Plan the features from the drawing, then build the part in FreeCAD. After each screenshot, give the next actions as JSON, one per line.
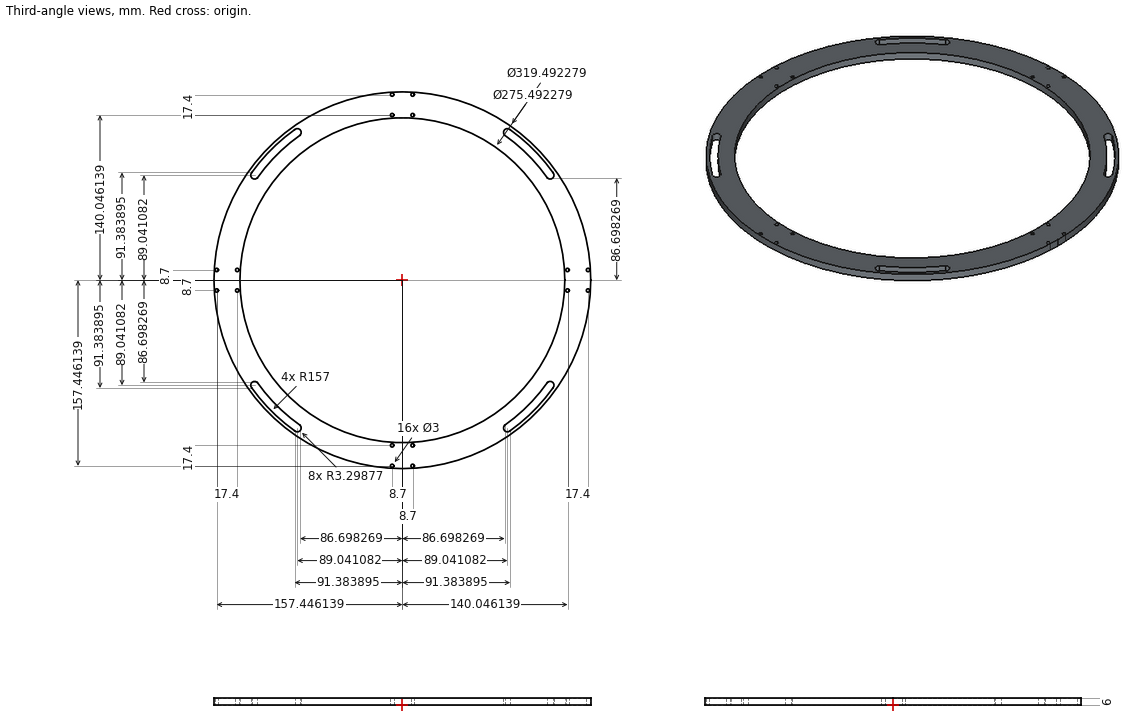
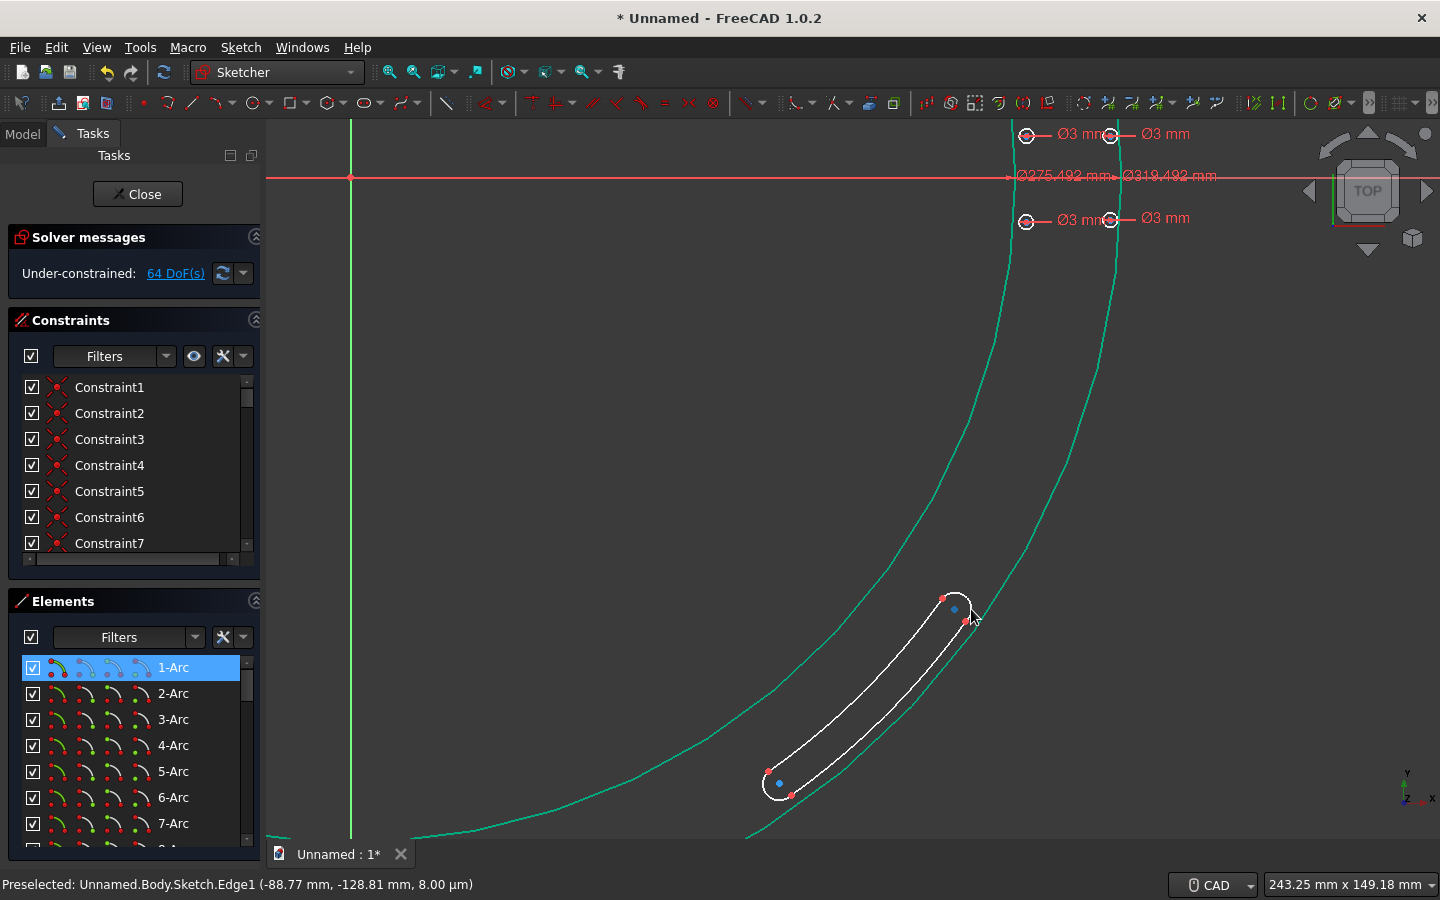
{"action": "left_click", "coordinate": [971, 607]}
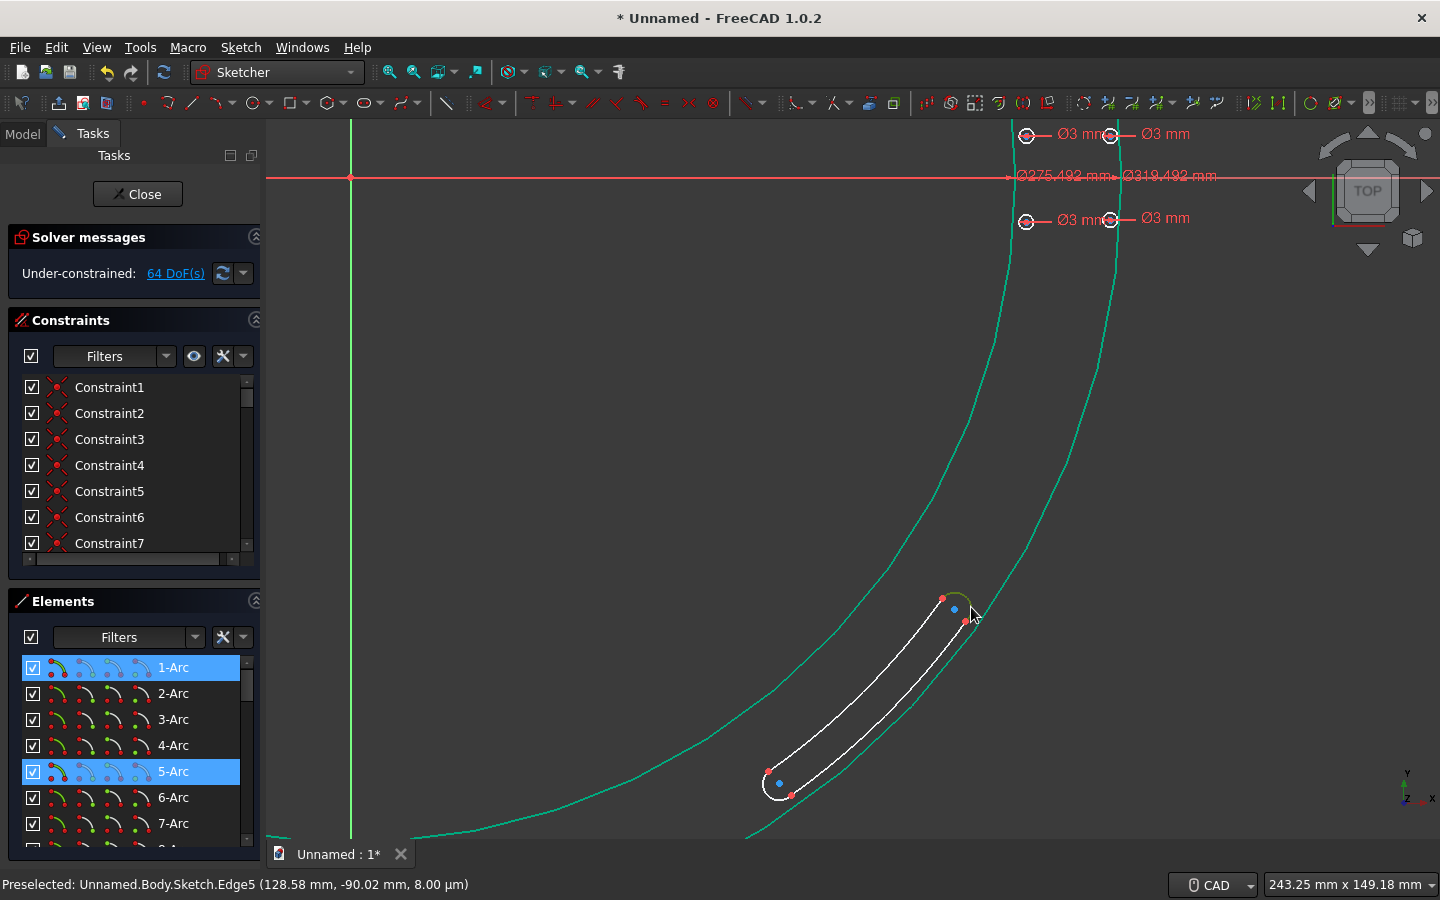
{"action": "scroll", "coordinate": [972, 609], "scroll_direction": "down", "scroll_amount": 6}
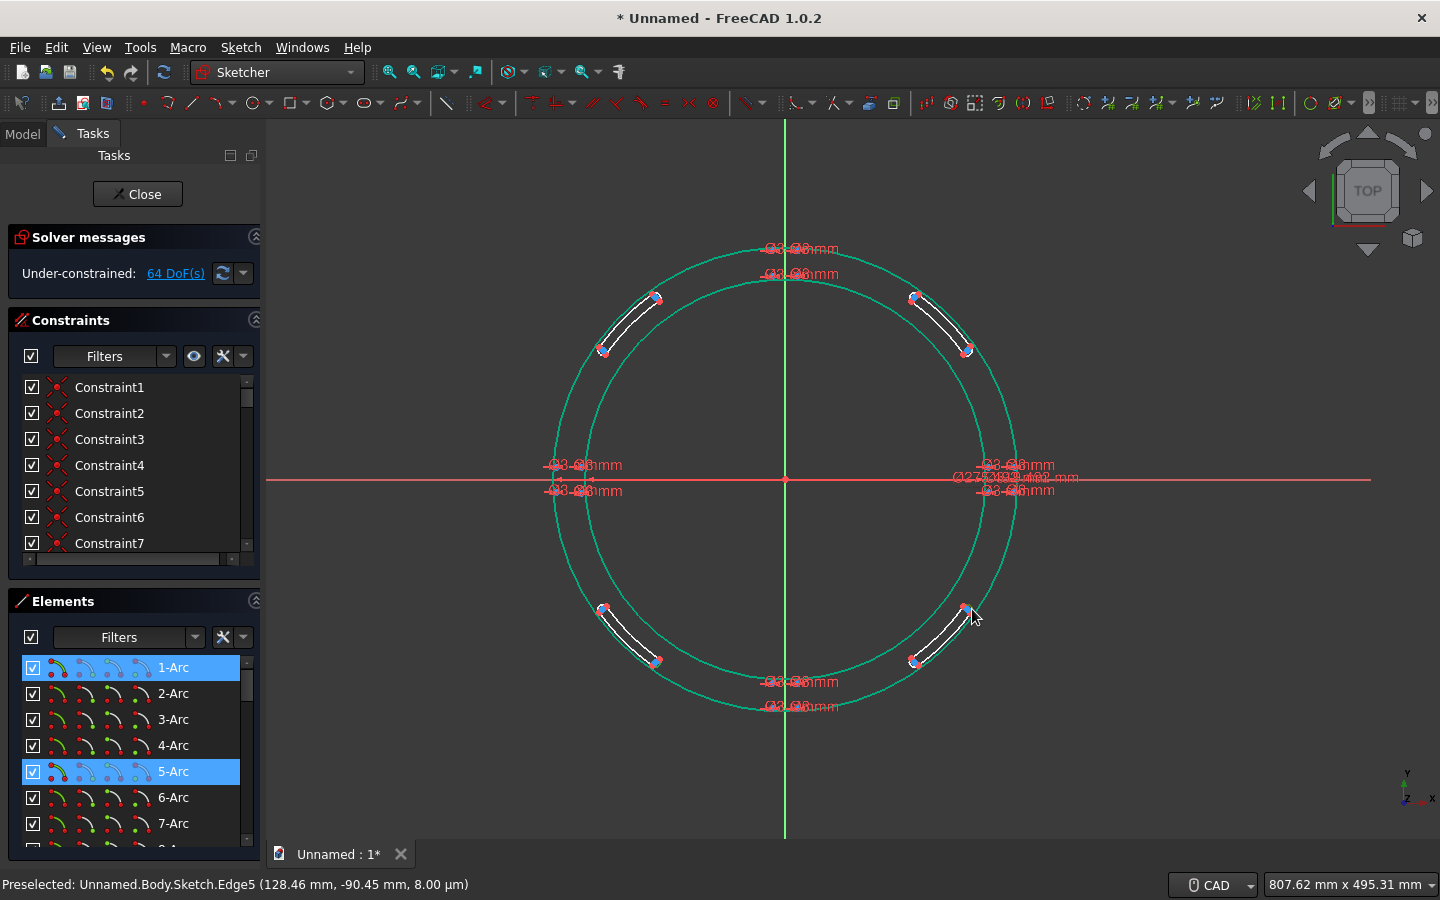
{"action": "scroll", "coordinate": [598, 352], "scroll_direction": "up", "scroll_amount": 7}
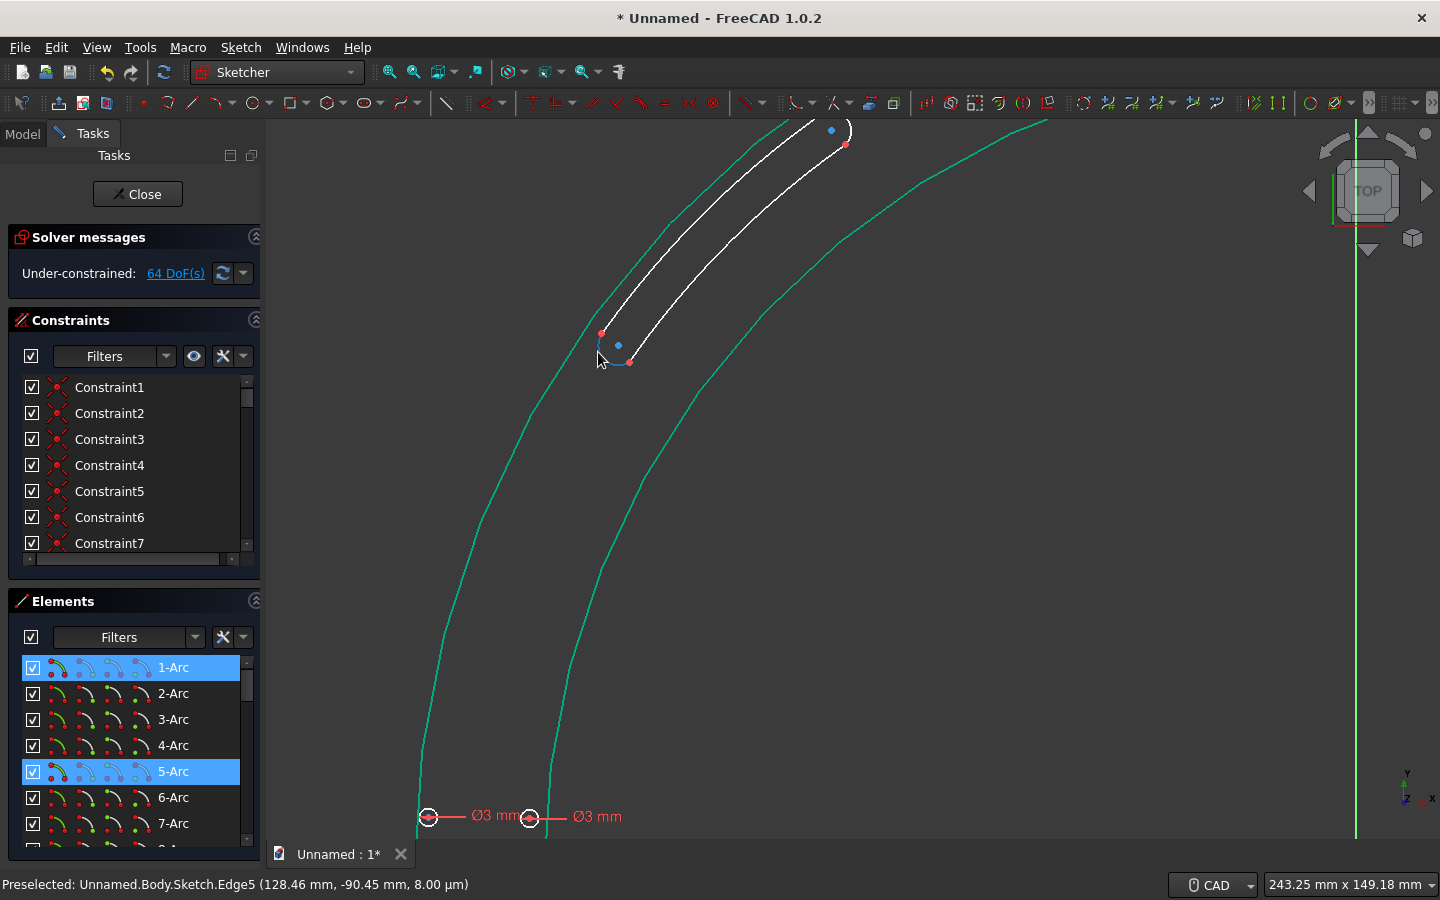
{"action": "left_click", "coordinate": [599, 350]}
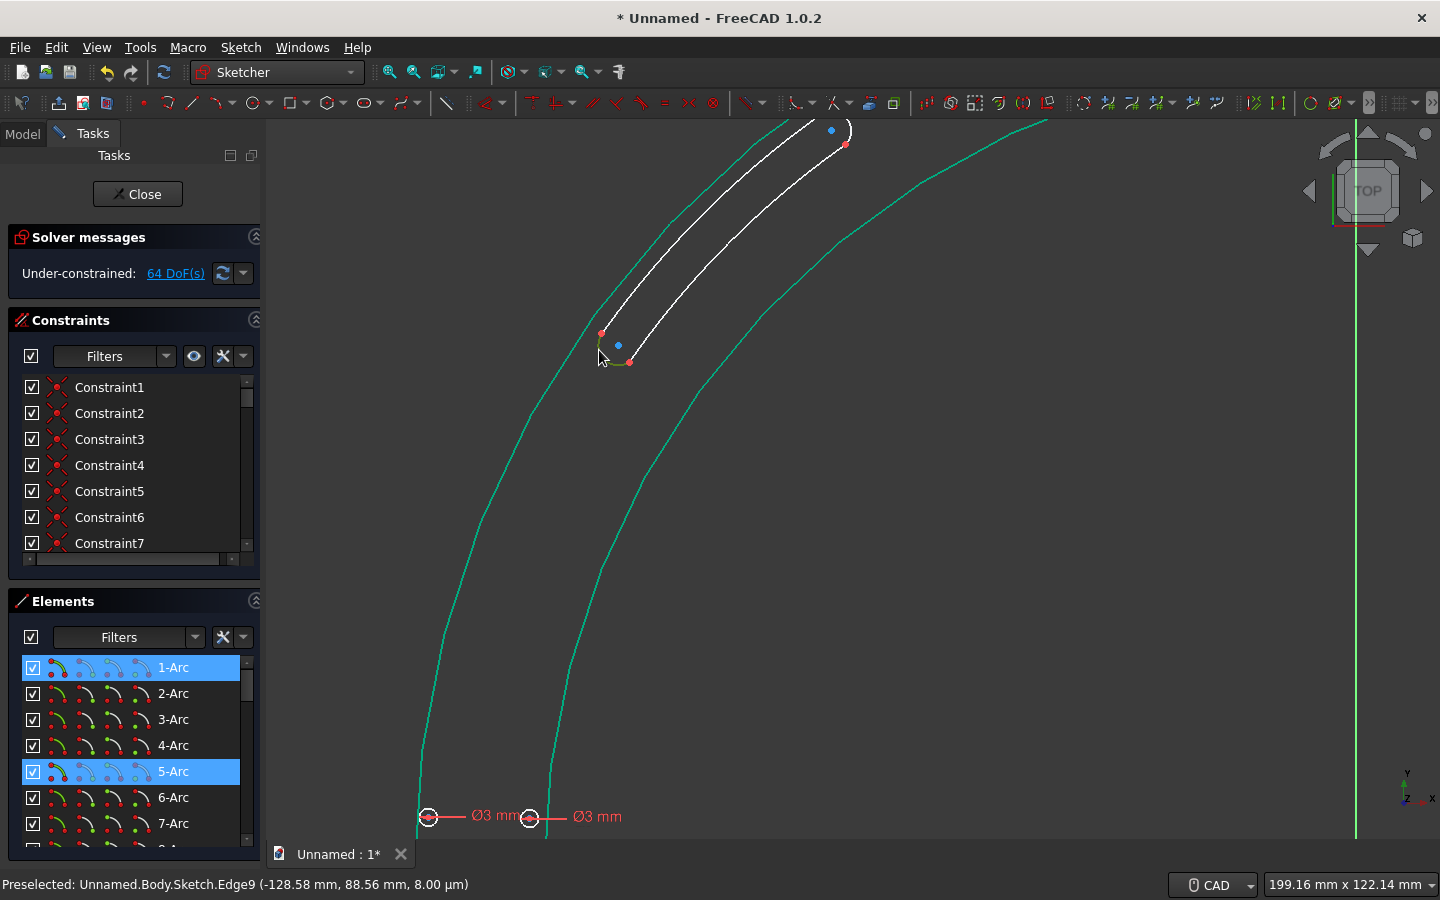
{"action": "scroll", "coordinate": [597, 352], "scroll_direction": "down", "scroll_amount": 7}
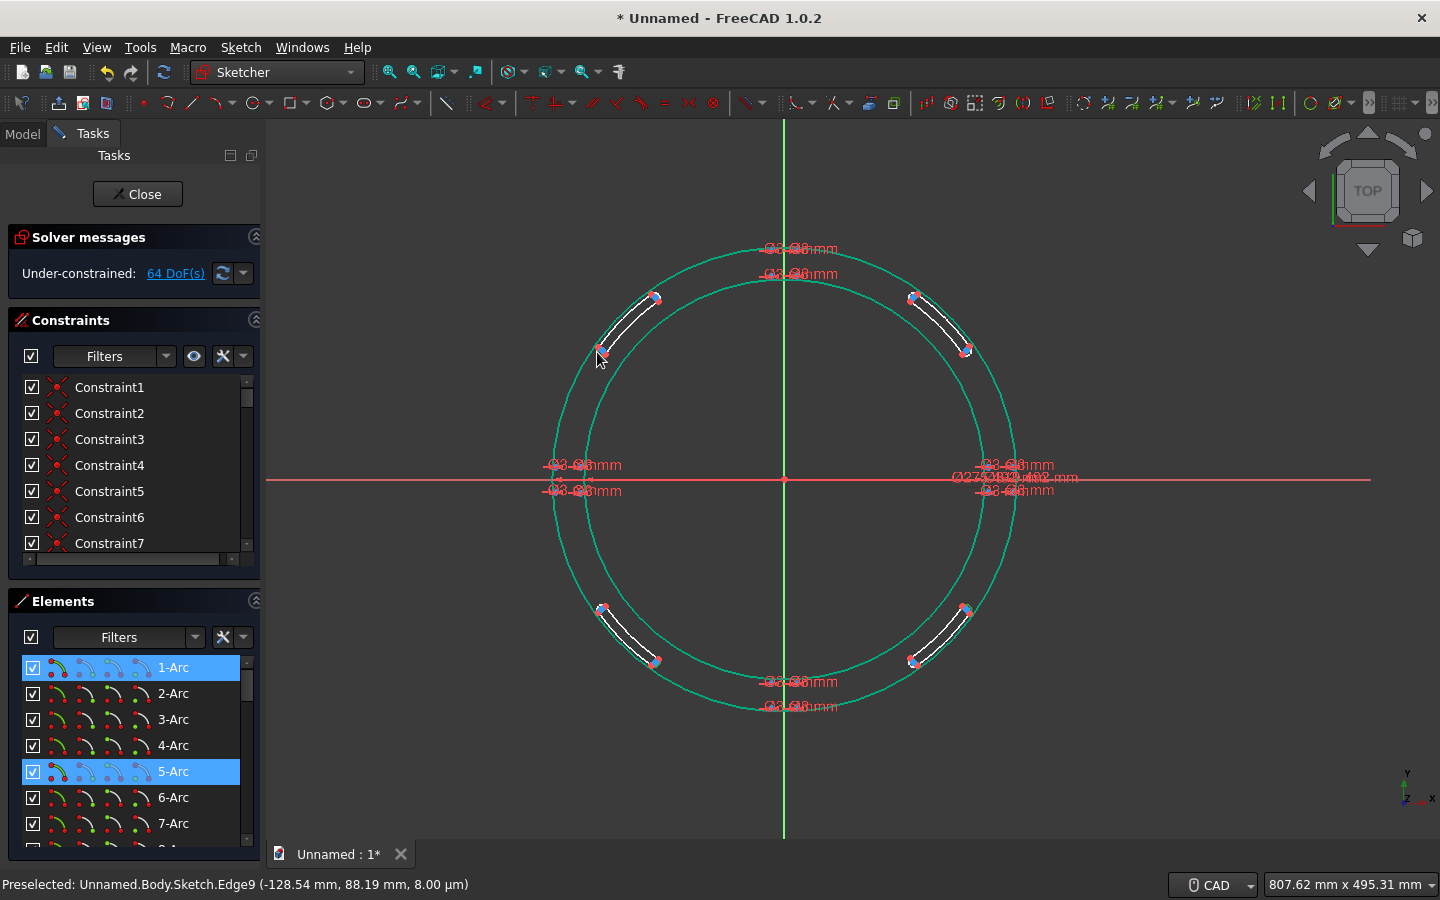
{"action": "scroll", "coordinate": [913, 293], "scroll_direction": "up", "scroll_amount": 6}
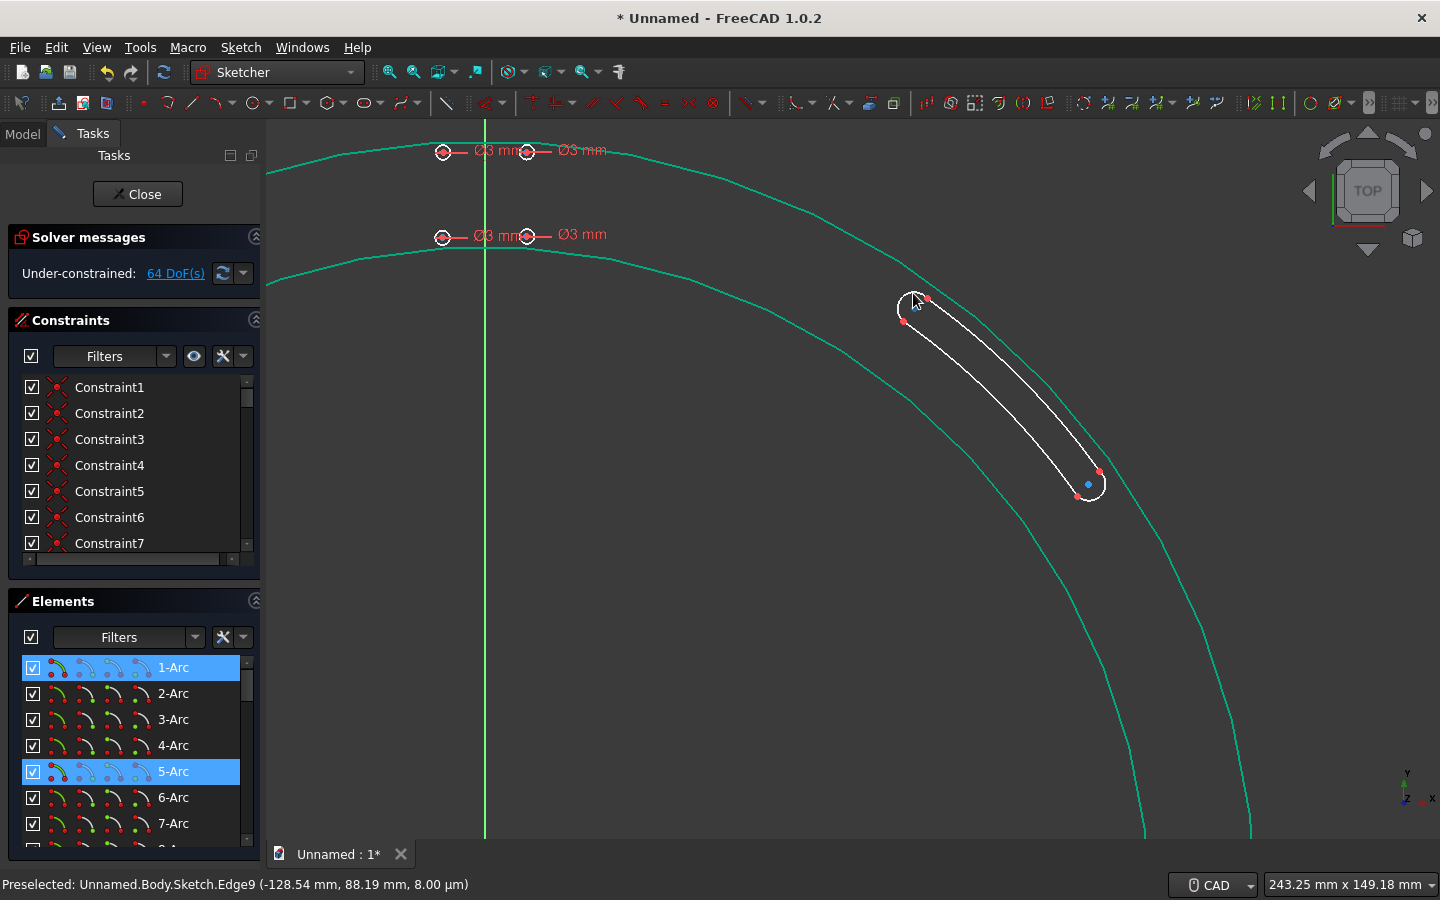
{"action": "left_click", "coordinate": [912, 292]}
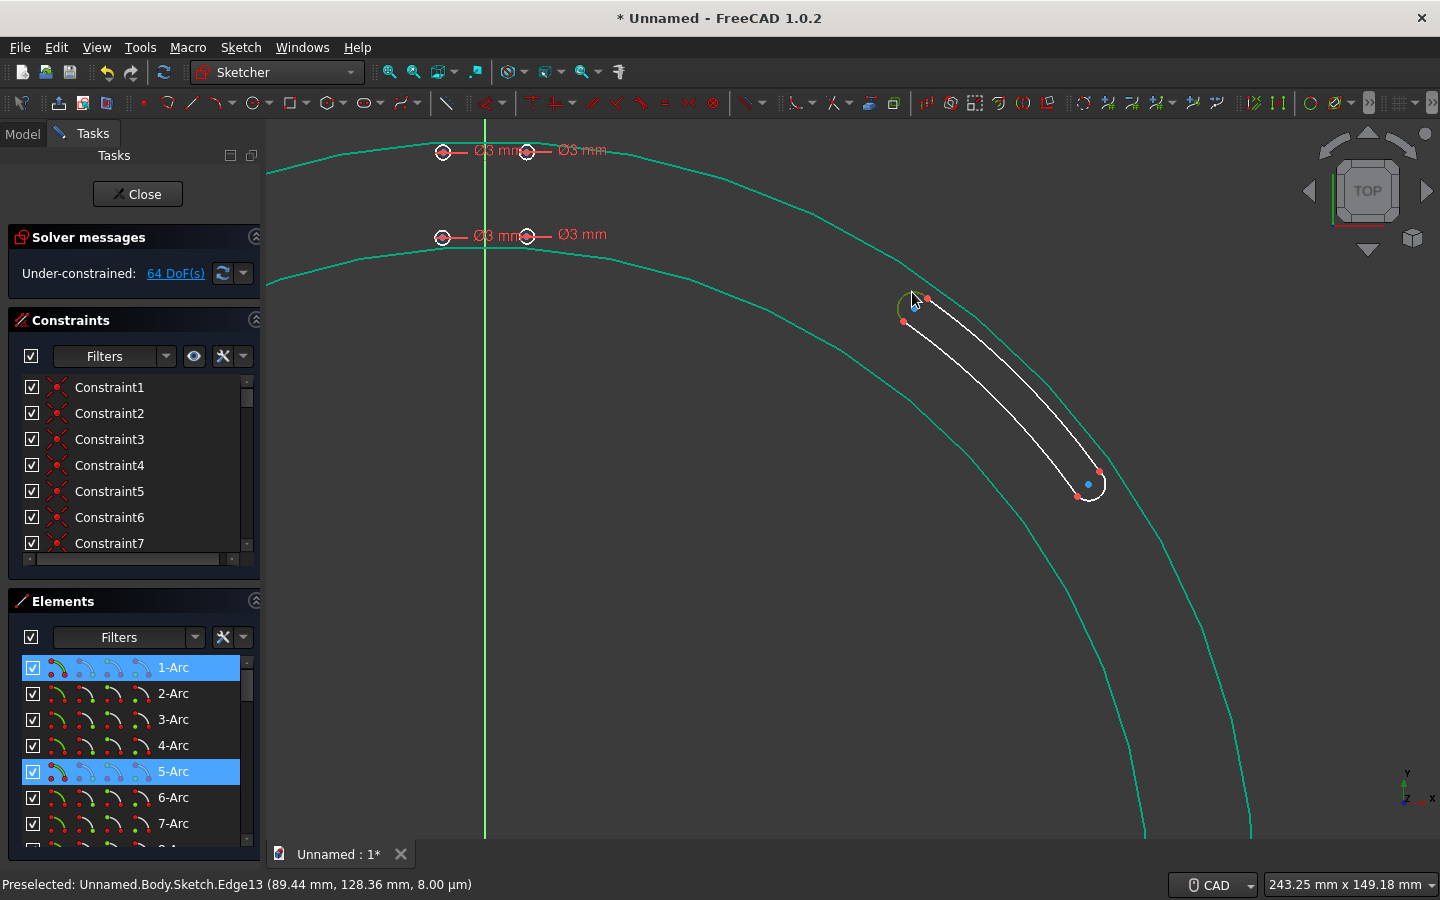
{"action": "key", "text": "e"}